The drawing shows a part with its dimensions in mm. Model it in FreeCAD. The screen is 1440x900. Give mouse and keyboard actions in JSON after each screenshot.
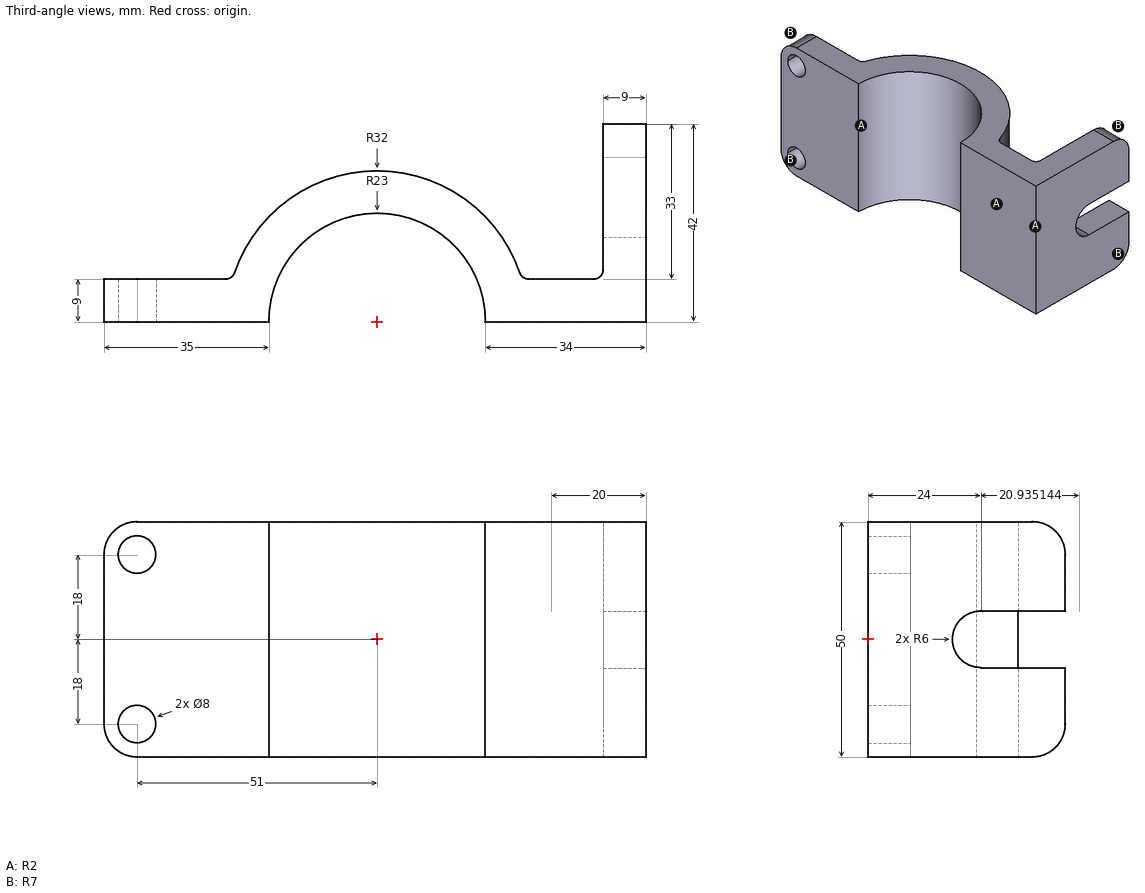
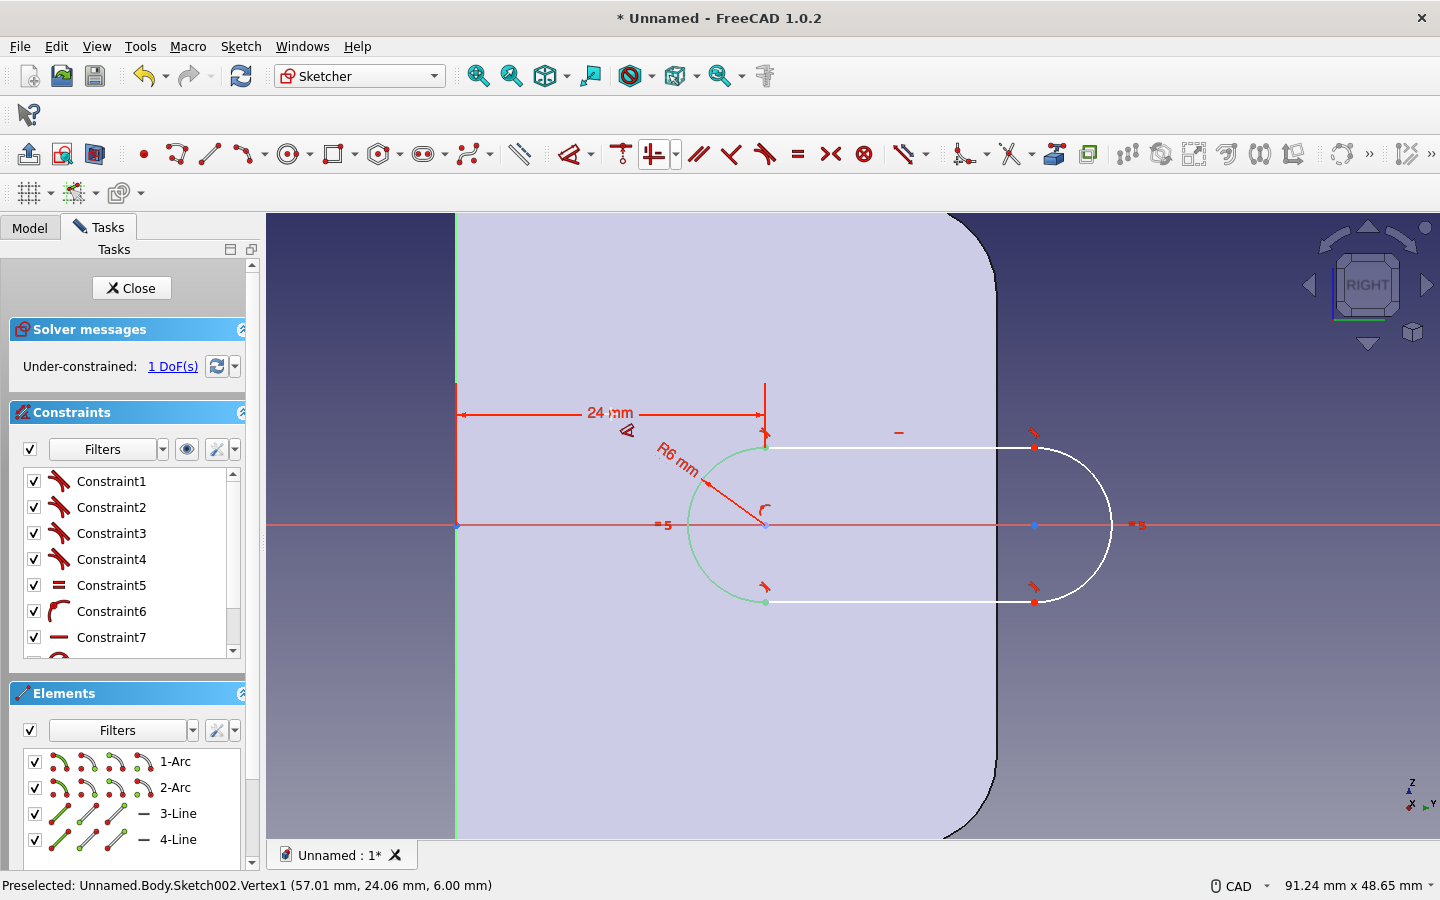
{"action": "left_click", "coordinate": [846, 448]}
{"action": "left_click", "coordinate": [900, 414]}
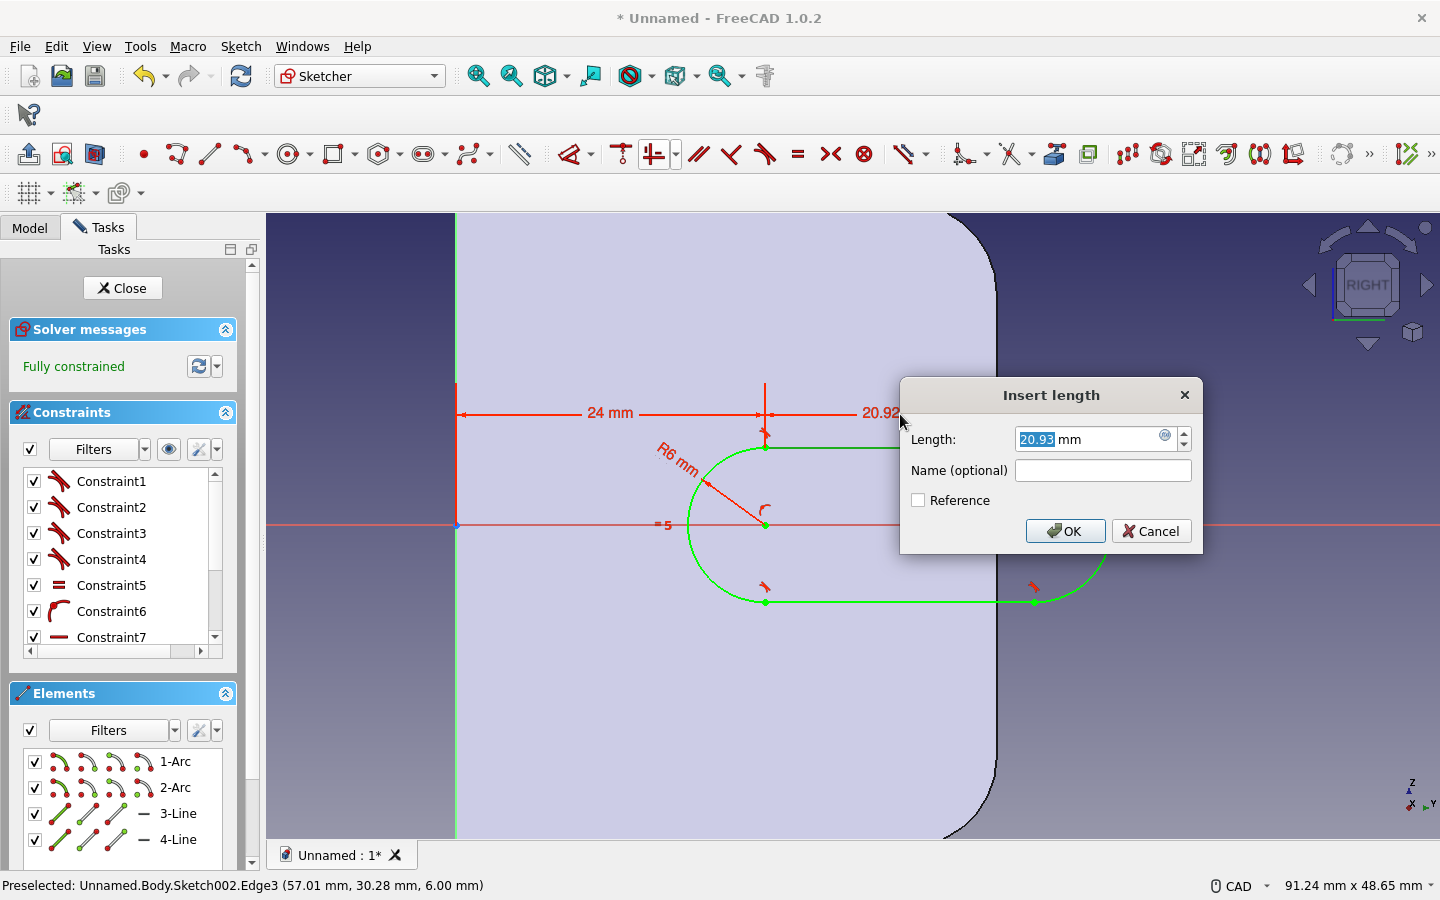
{"action": "type", "text": "20.935144"}
{"action": "key", "text": "Return"}
{"action": "key", "text": "Escape"}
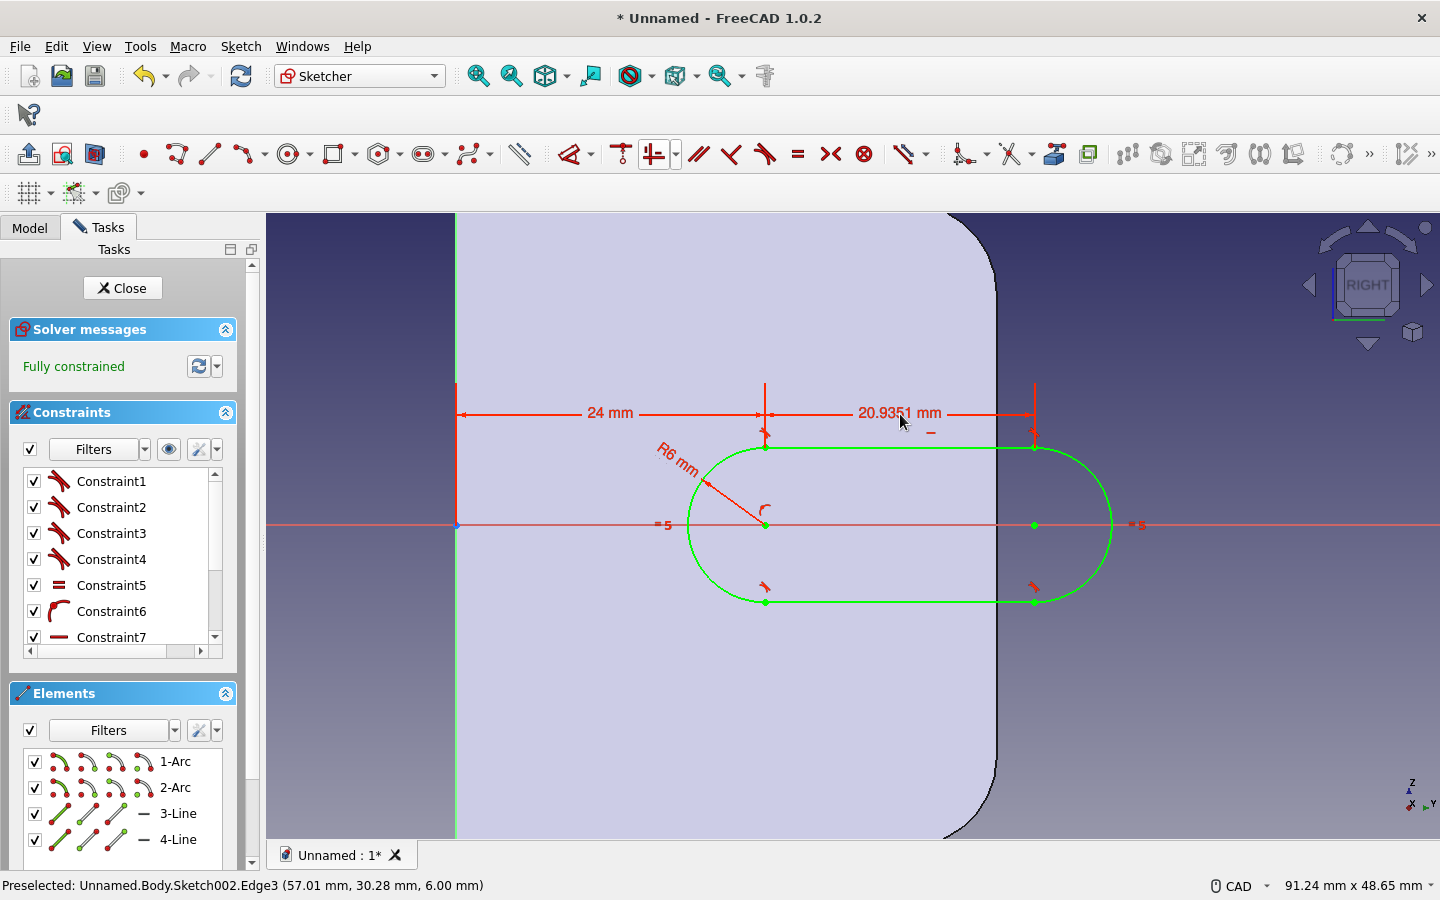
{"action": "left_click", "coordinate": [123, 288]}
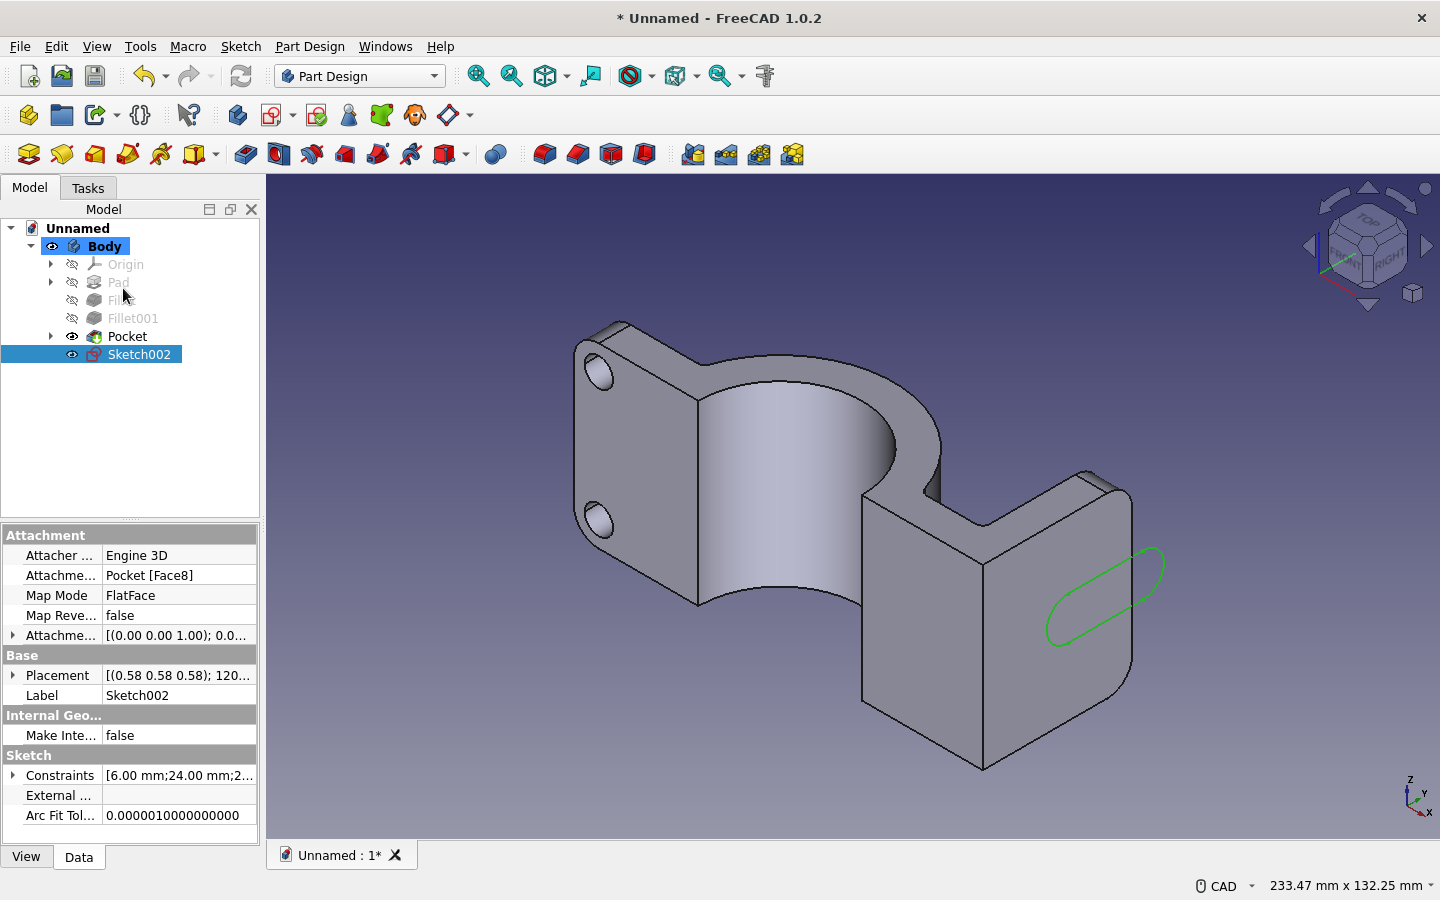
{"action": "left_click", "coordinate": [246, 154]}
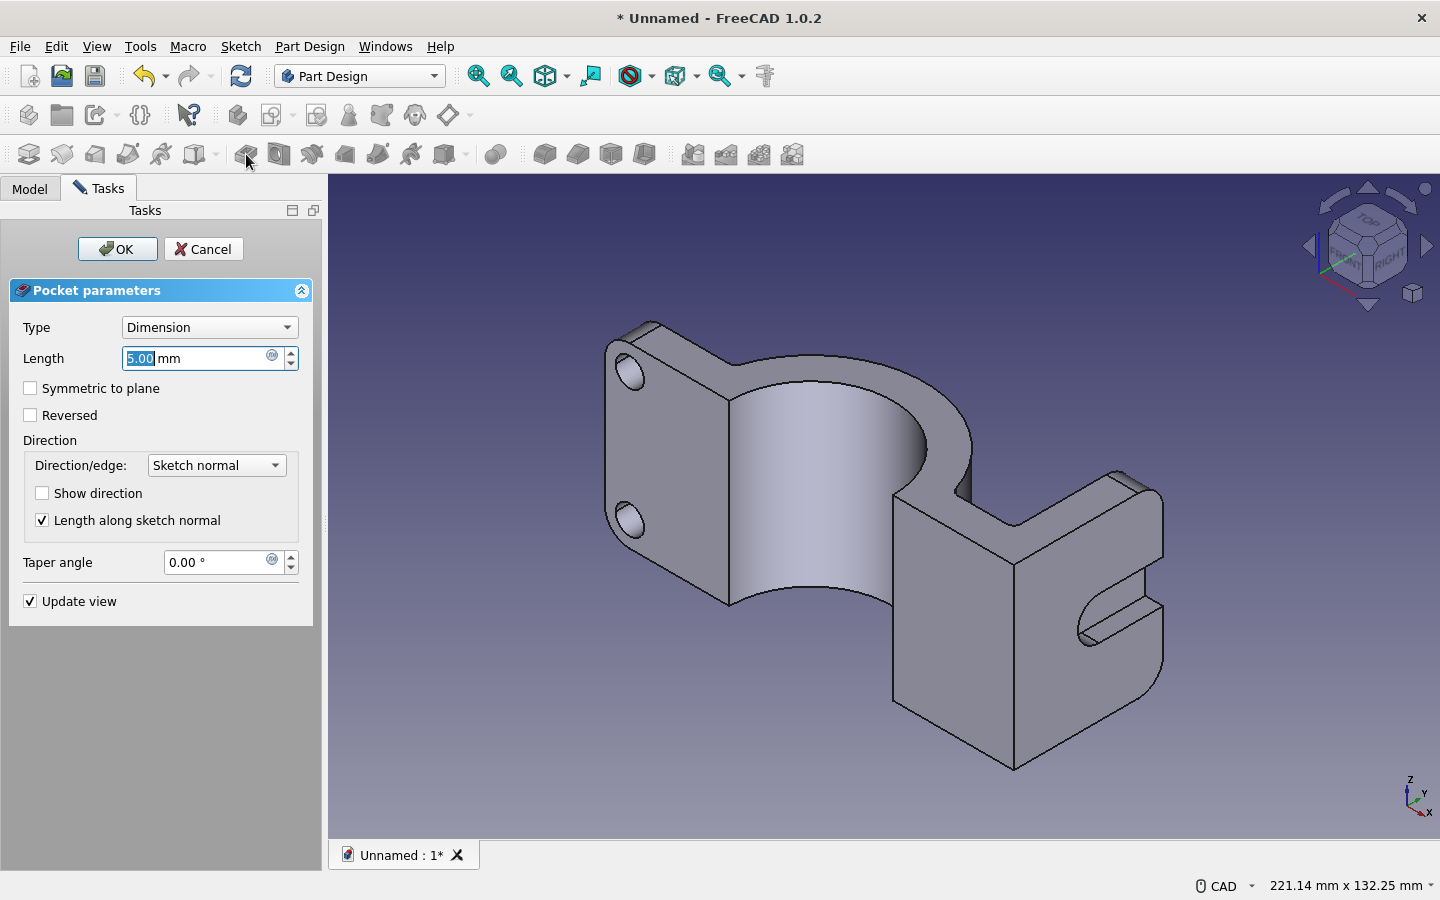
{"action": "type", "text": "20"}
{"action": "key", "text": "Tab"}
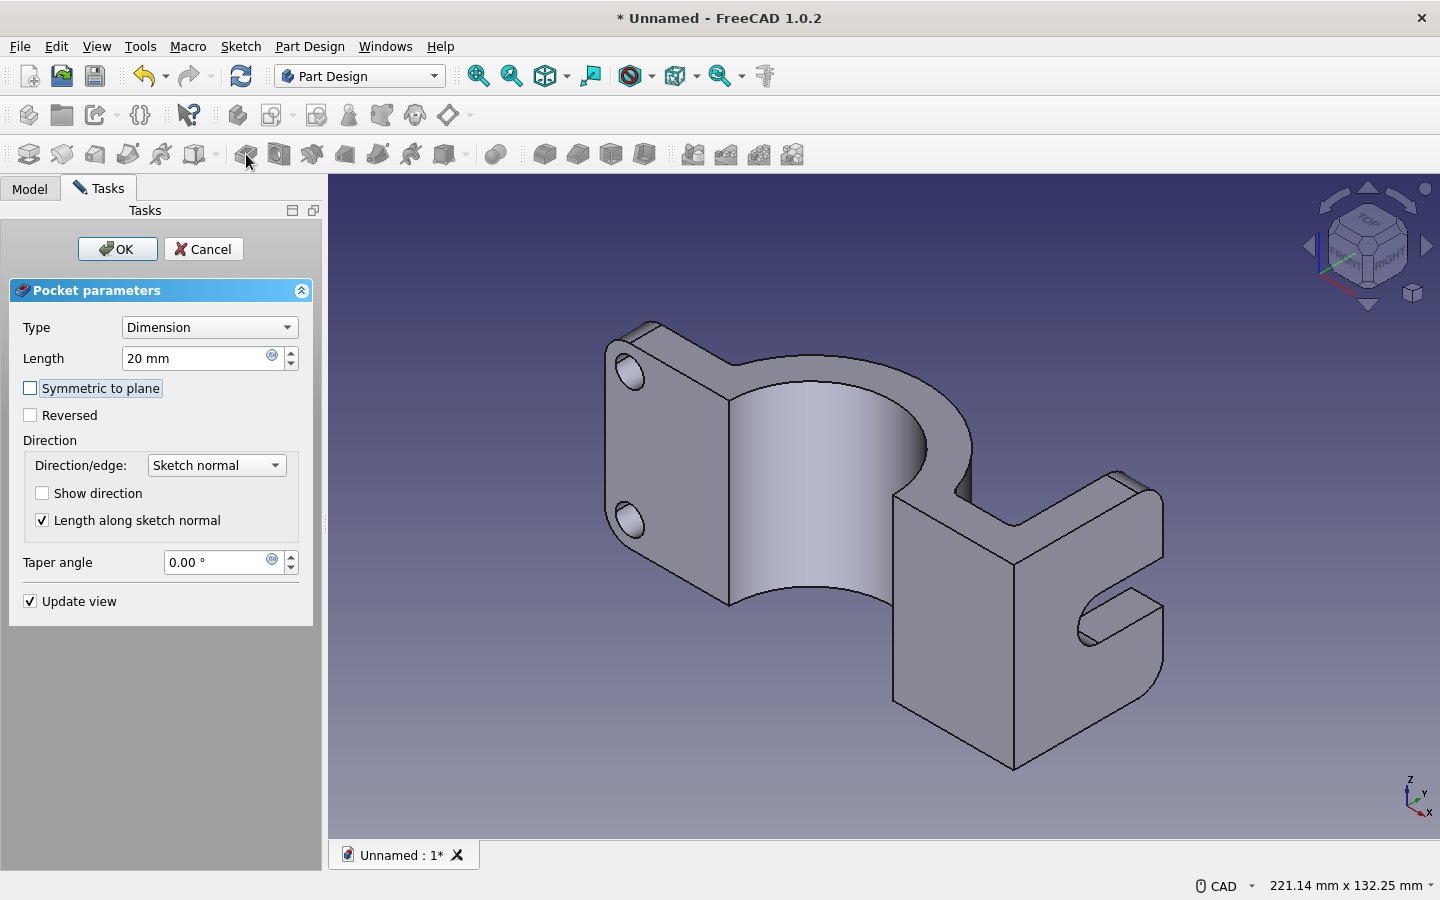
{"action": "left_click", "coordinate": [118, 249]}